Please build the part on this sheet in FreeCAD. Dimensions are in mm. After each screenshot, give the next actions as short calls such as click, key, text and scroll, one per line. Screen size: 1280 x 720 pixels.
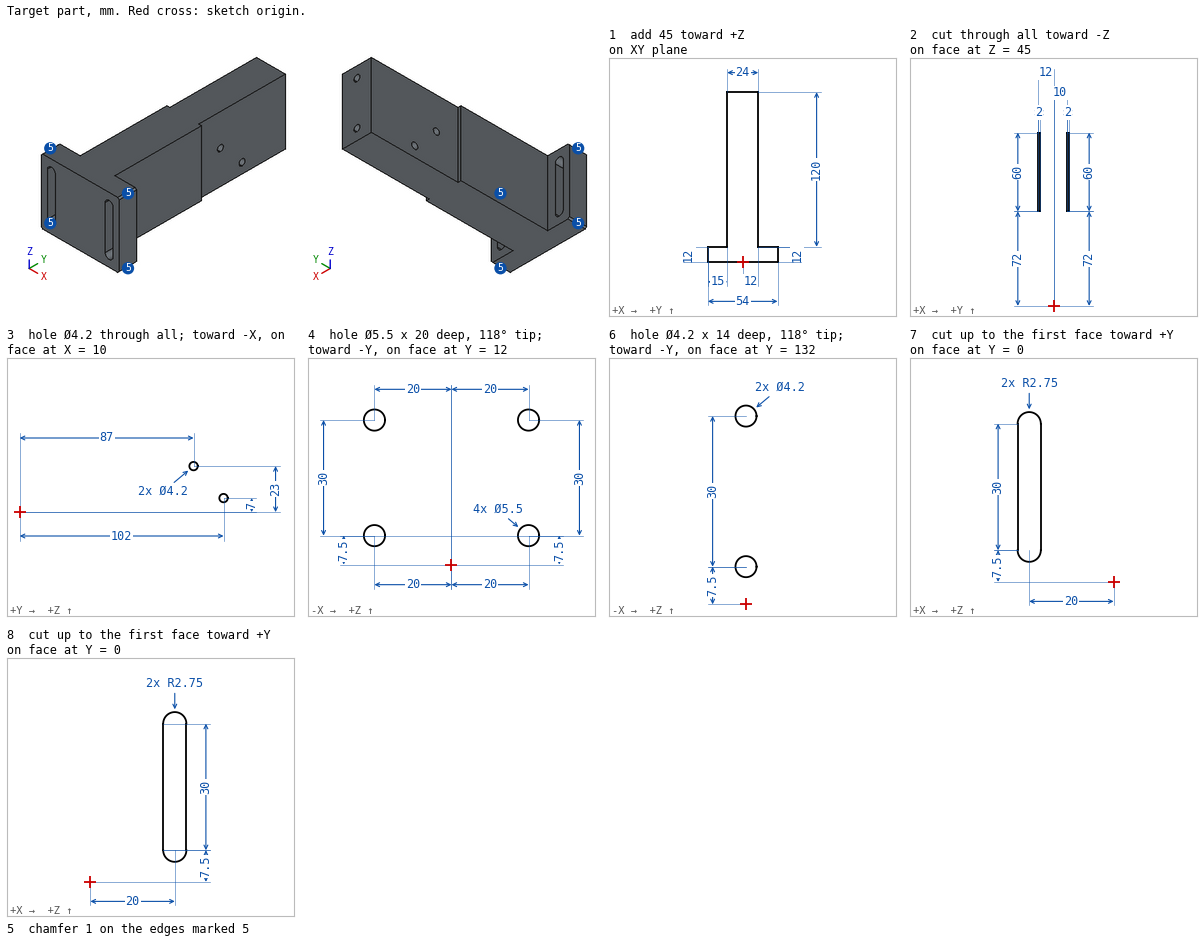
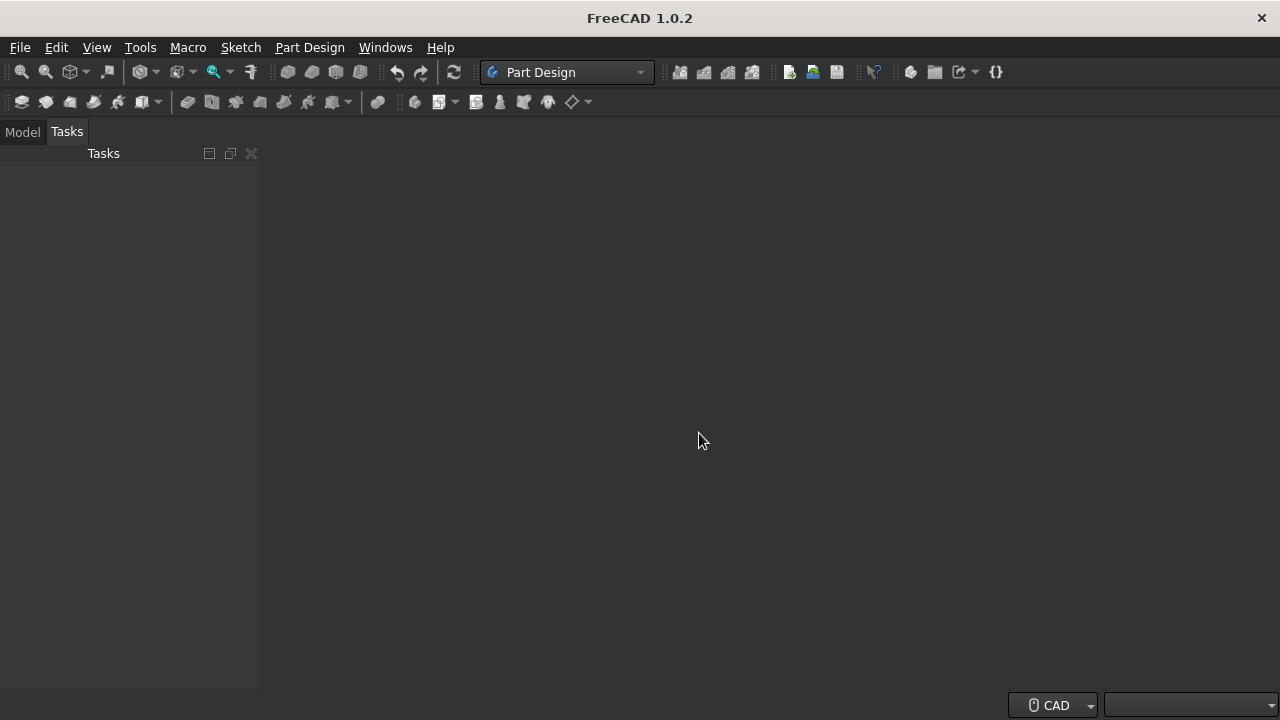
click(790, 72)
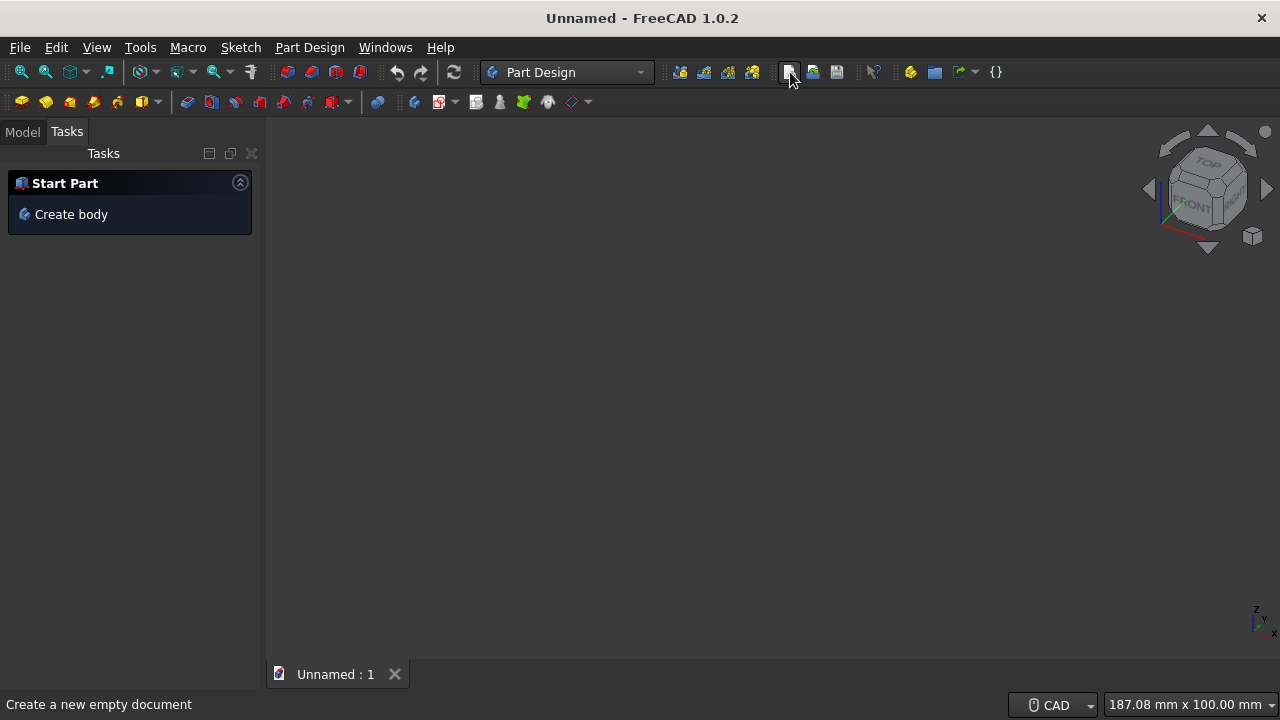
click(440, 102)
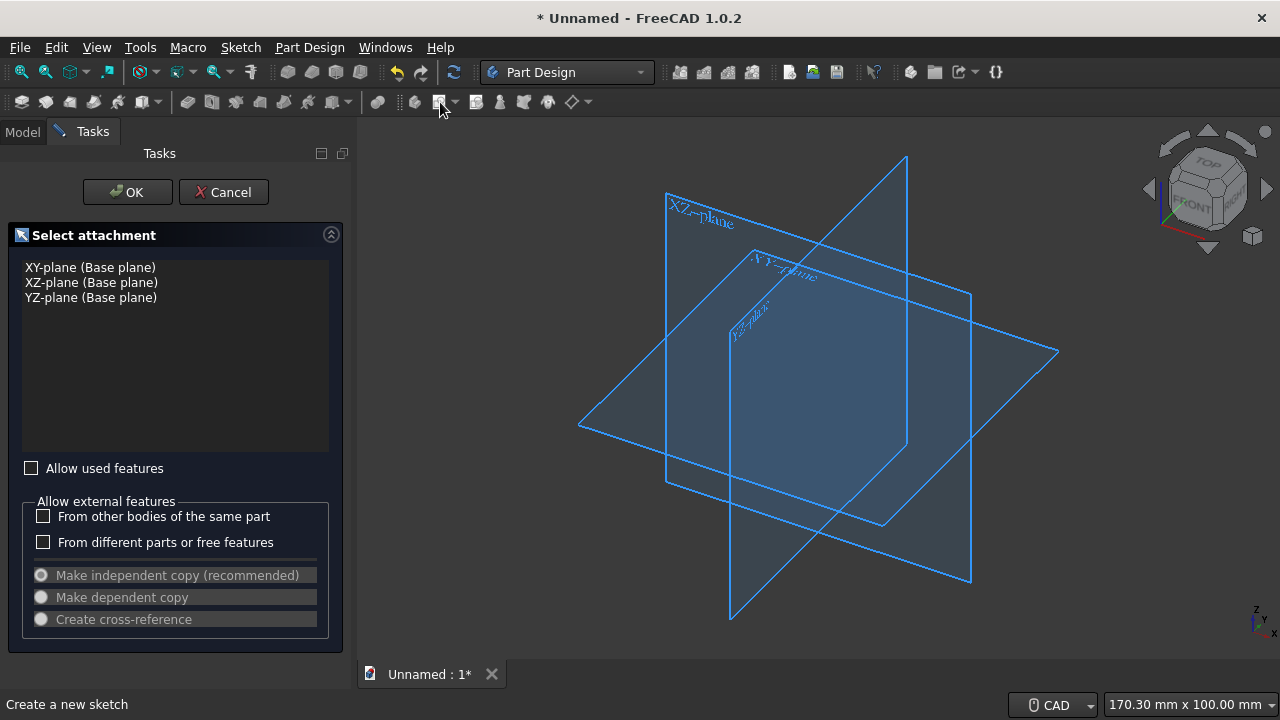
click(82, 268)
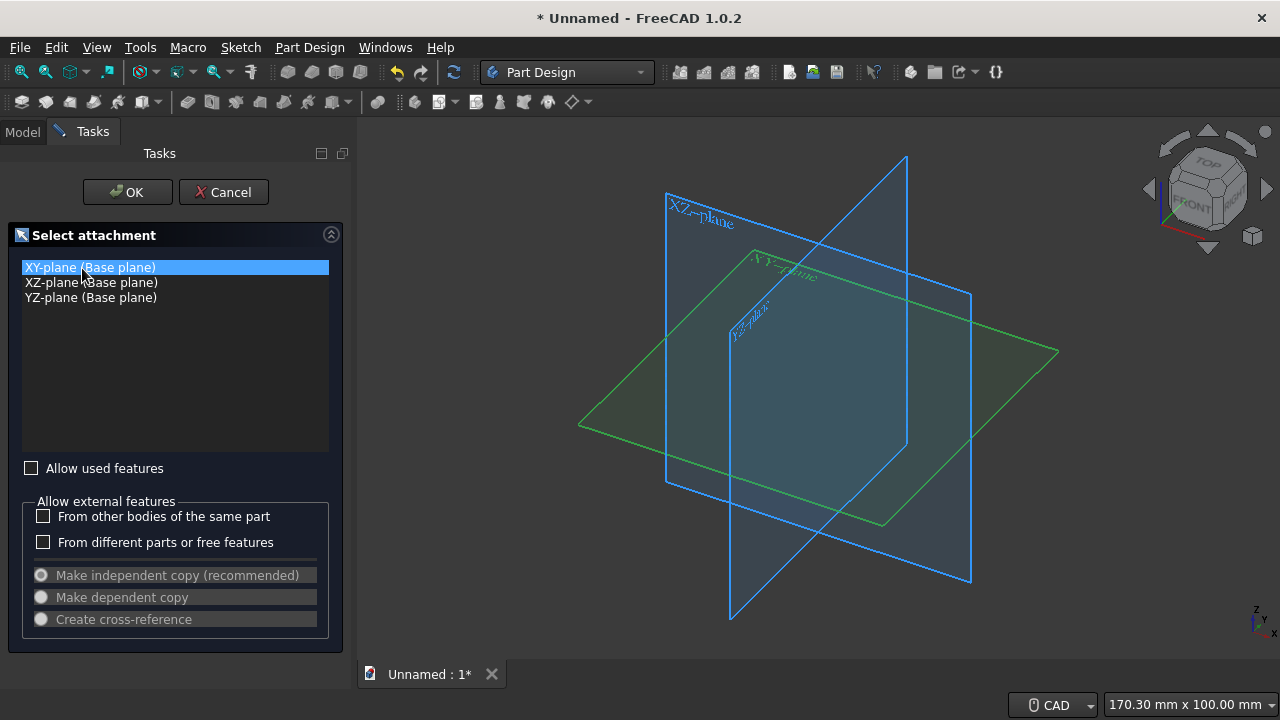
click(128, 192)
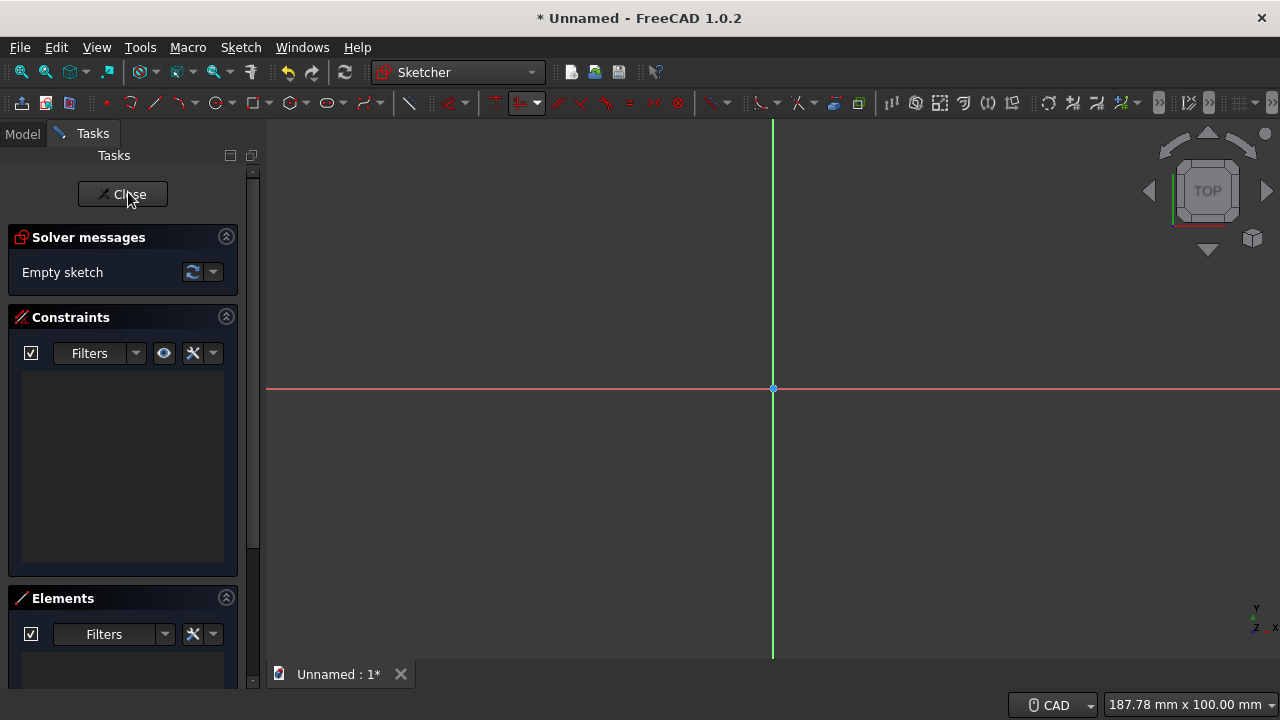
scroll(649, 631, down, 4)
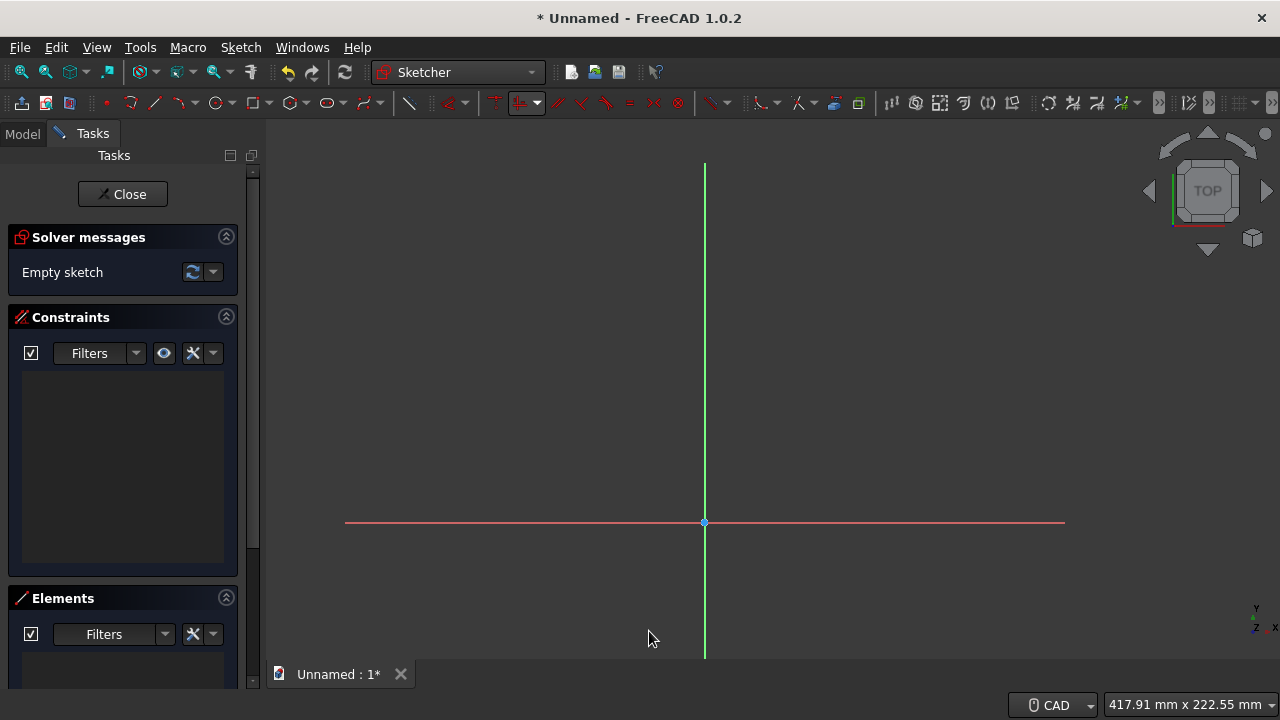
click(132, 104)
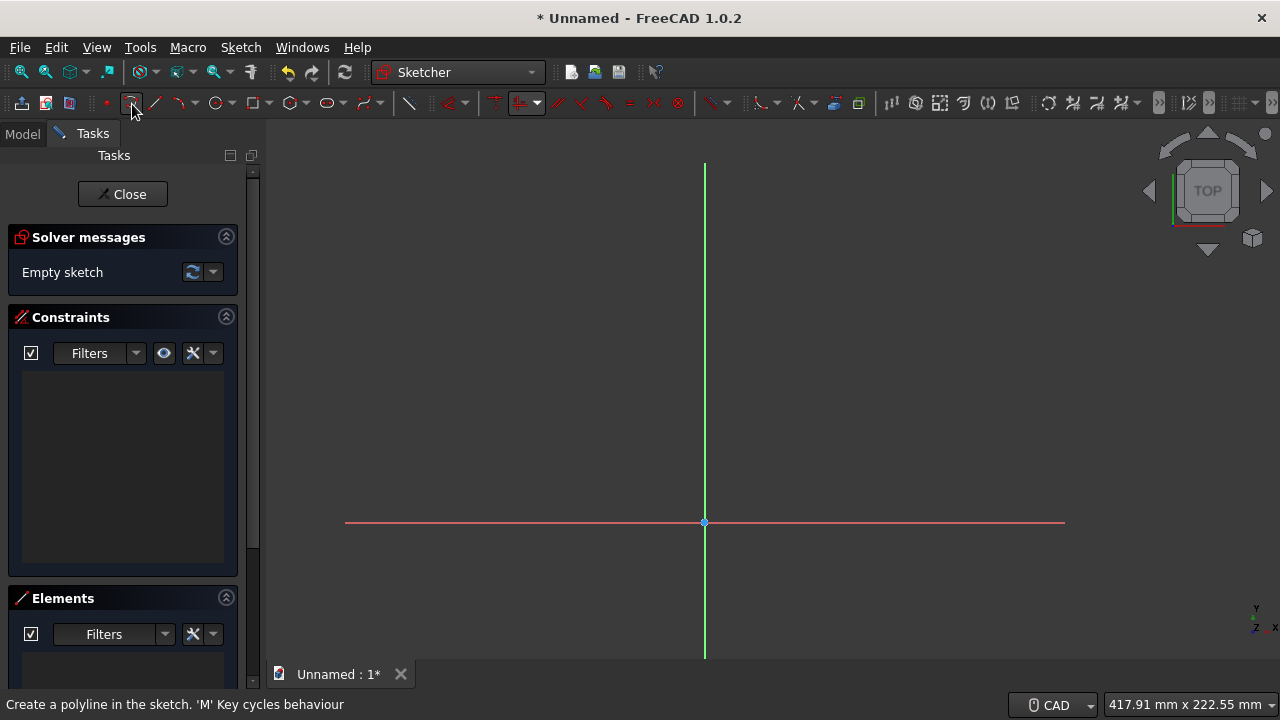
click(734, 494)
click(734, 203)
click(676, 203)
click(676, 494)
click(639, 494)
click(639, 523)
click(770, 514)
click(770, 494)
click(734, 495)
key(Escape)
key(Escape)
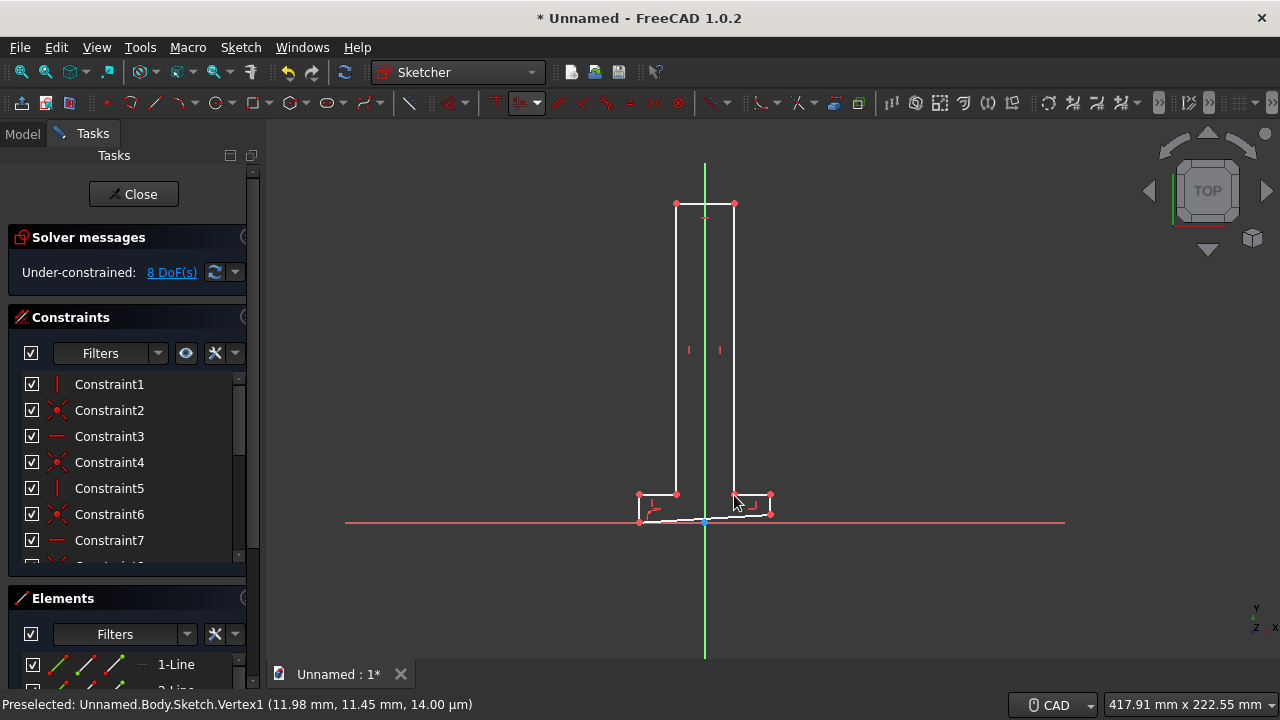
click(678, 520)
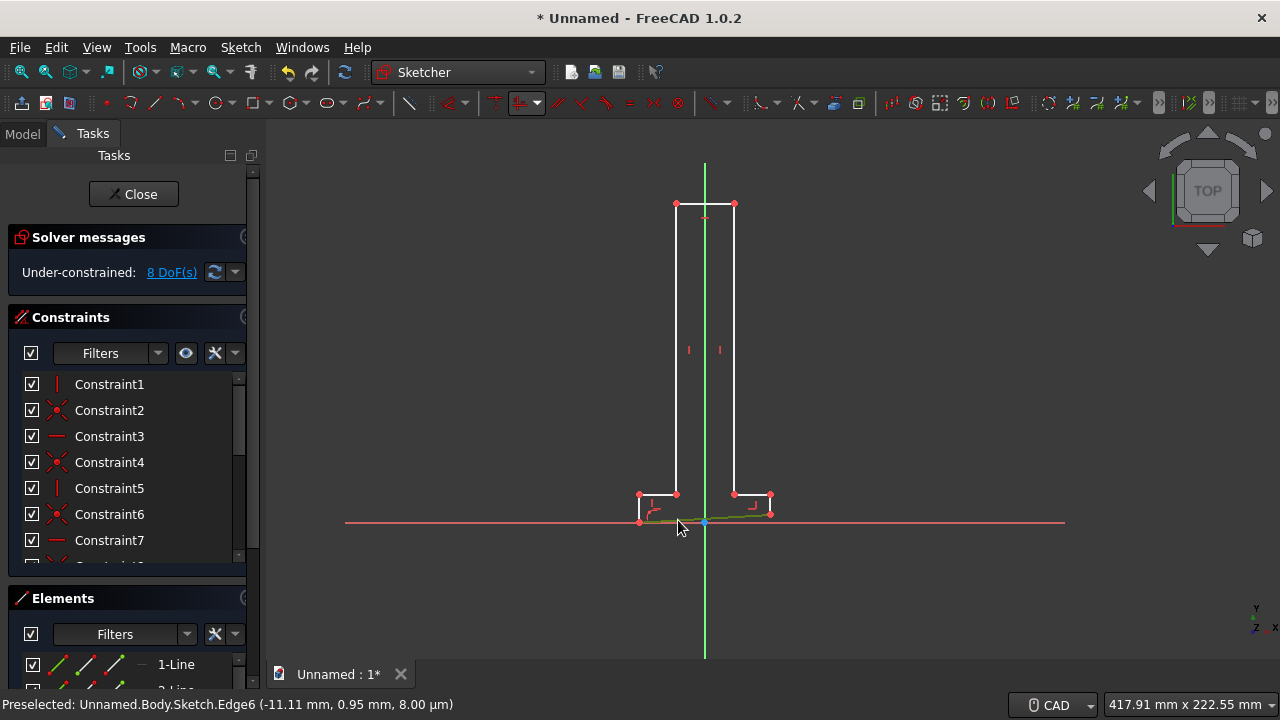
key(h)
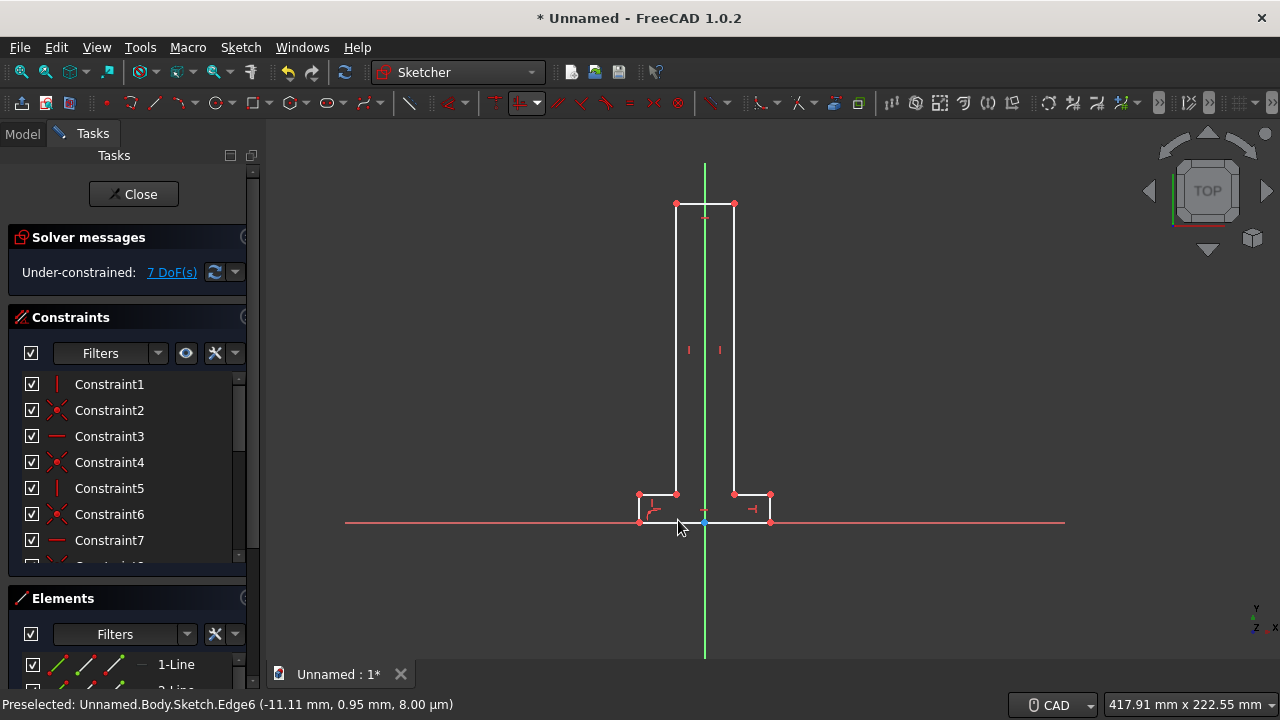
click(448, 104)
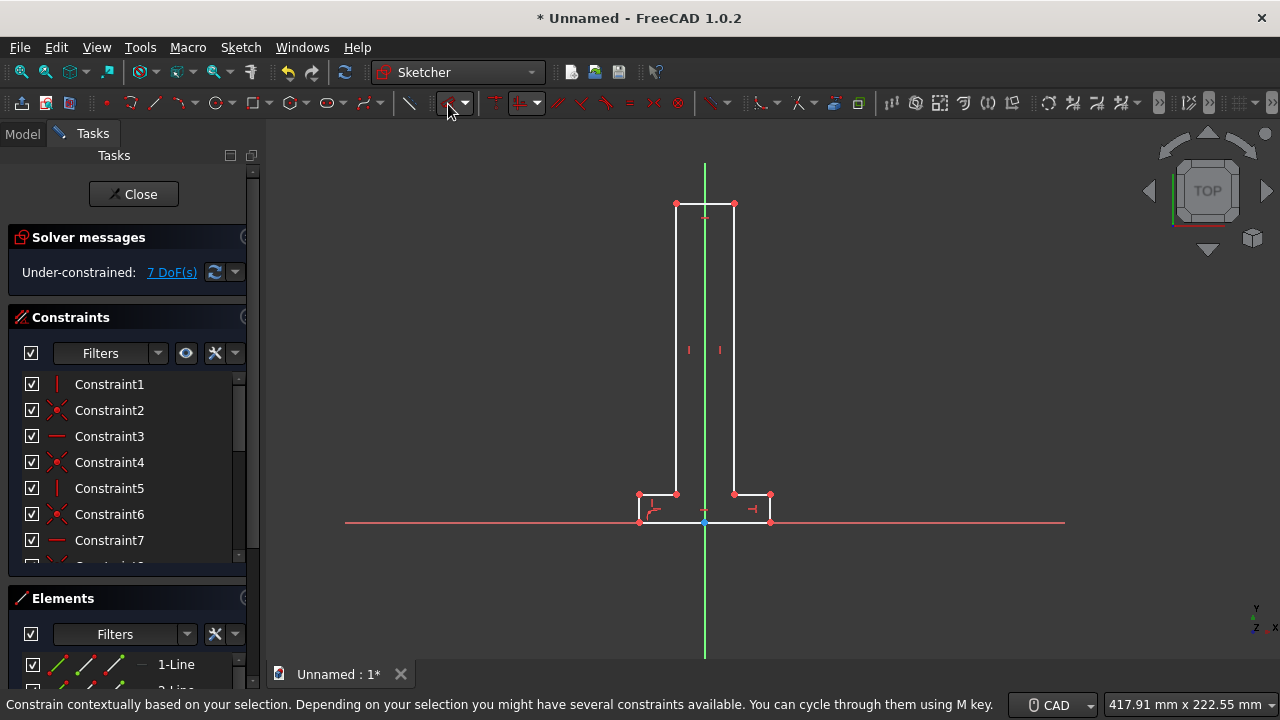
click(717, 204)
click(692, 170)